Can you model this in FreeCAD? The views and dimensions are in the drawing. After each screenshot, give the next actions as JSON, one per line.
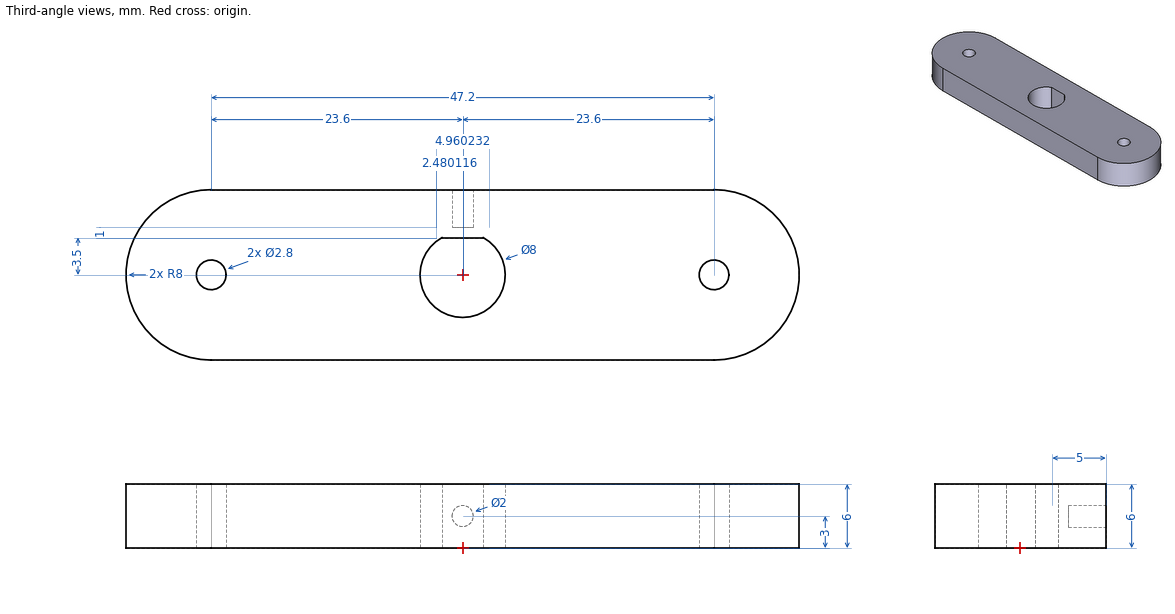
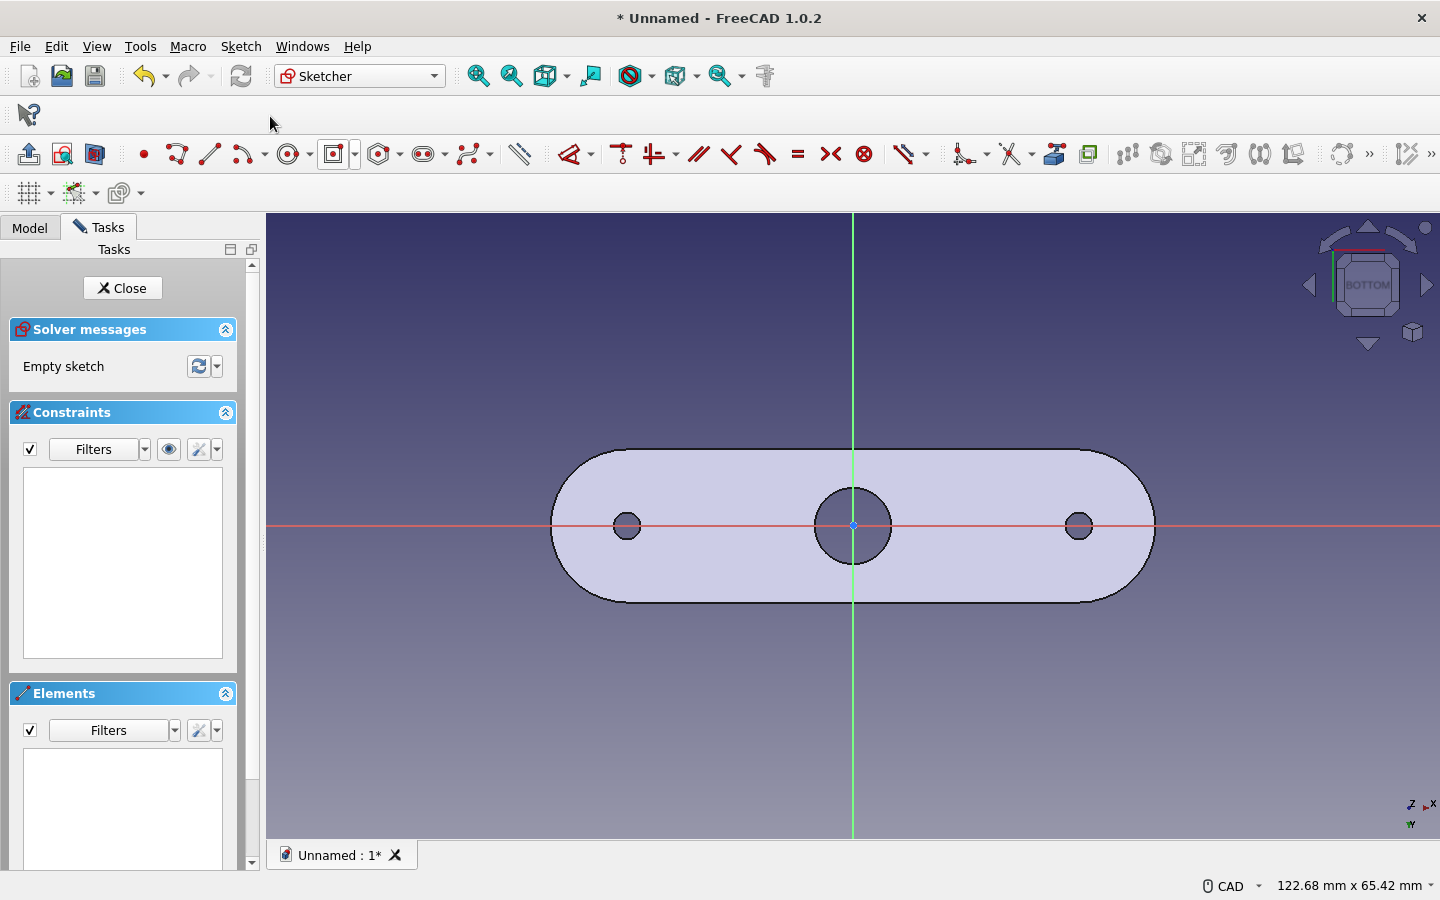
{"action": "scroll", "coordinate": [862, 550], "scroll_direction": "up", "scroll_amount": 11}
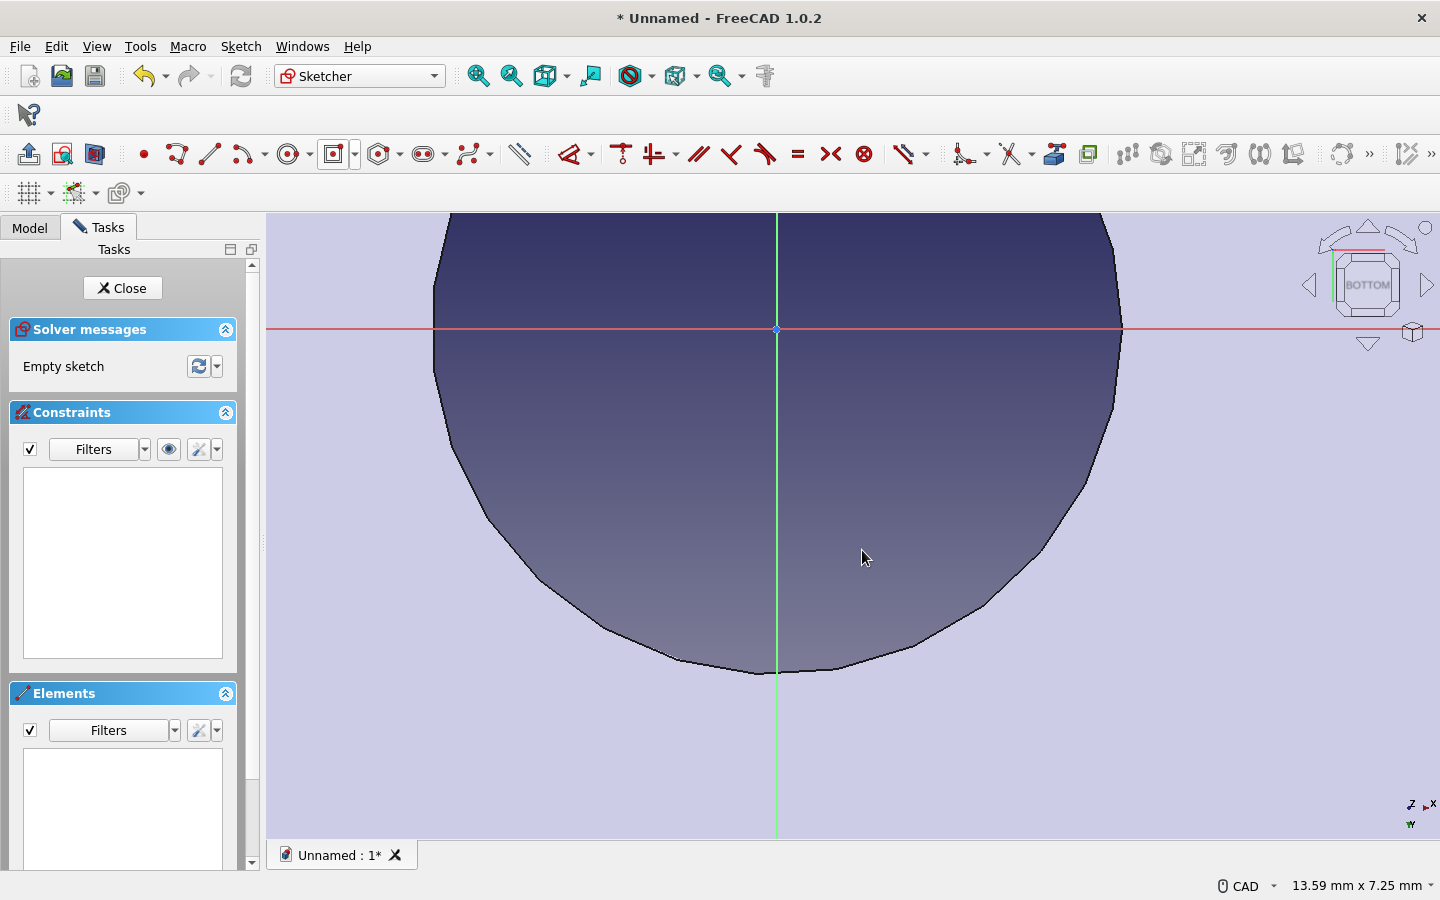
{"action": "left_click", "coordinate": [354, 154]}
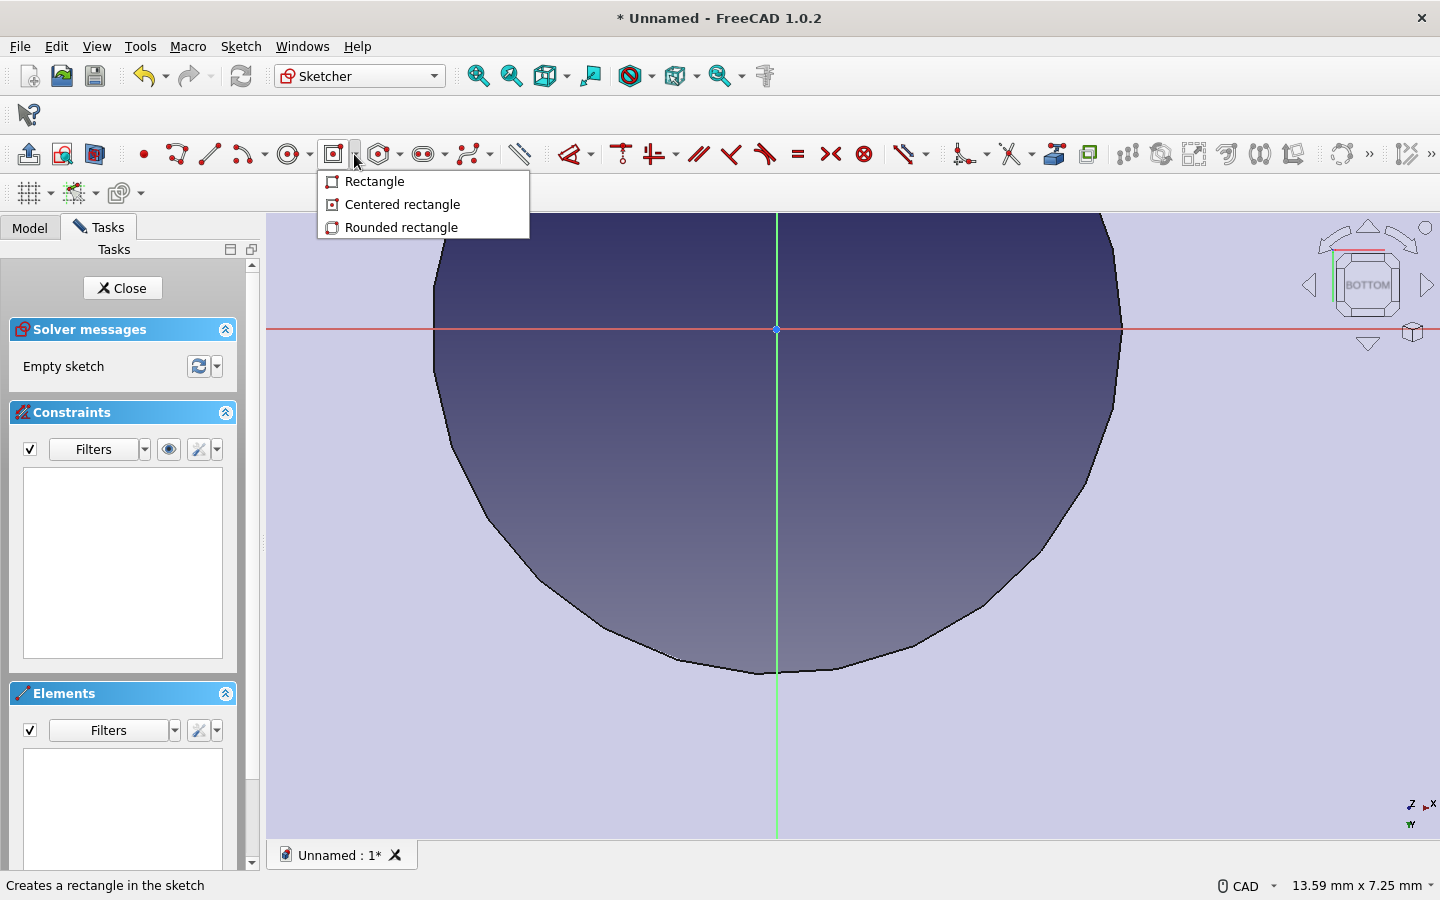
{"action": "left_click", "coordinate": [424, 182]}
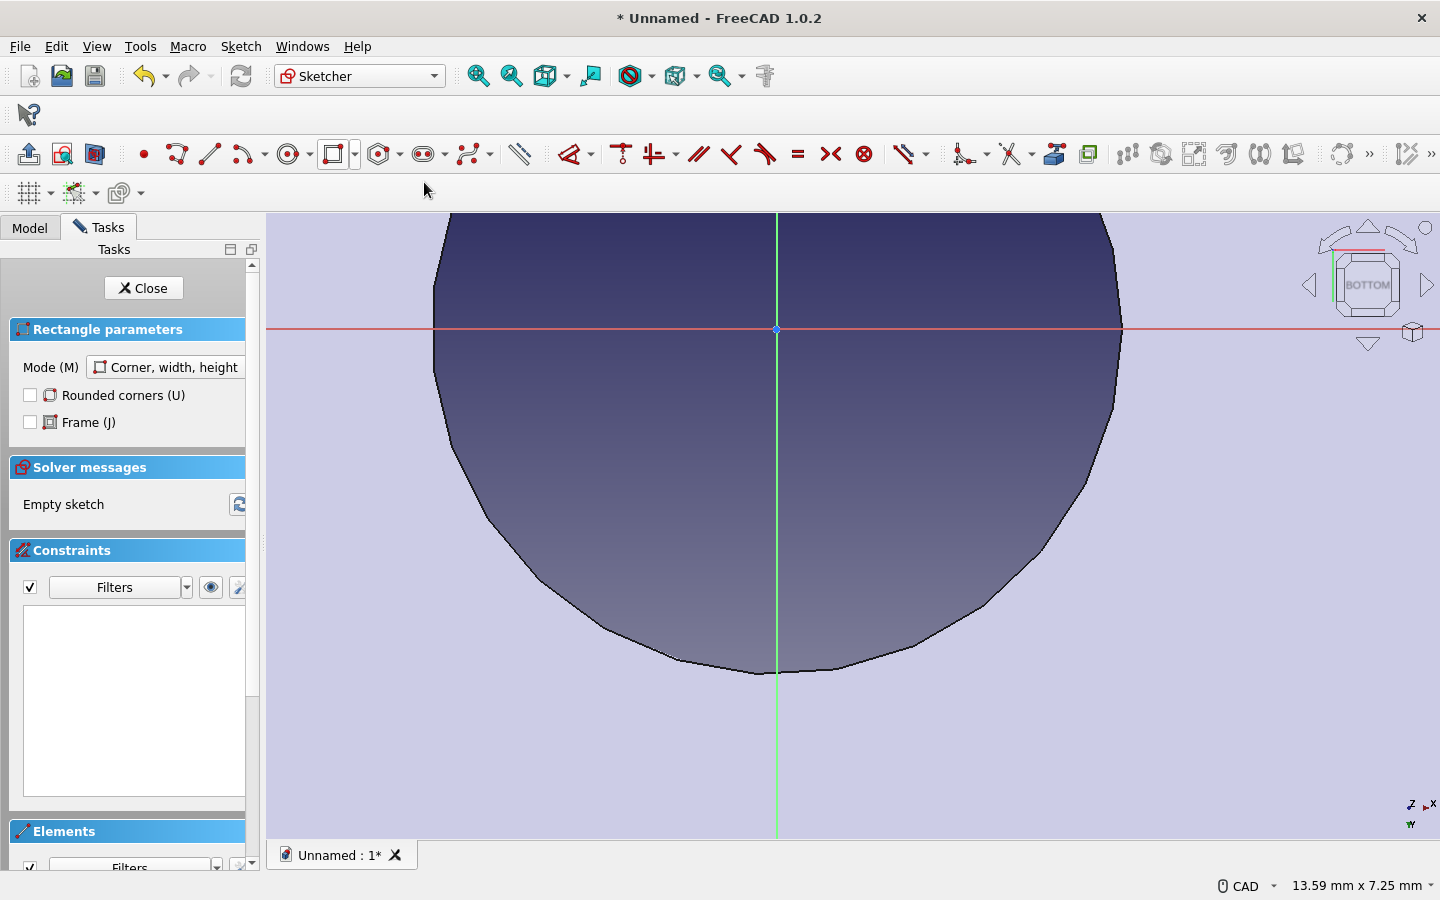
{"action": "left_click", "coordinate": [563, 631]}
{"action": "left_click", "coordinate": [991, 718]}
{"action": "key", "text": "Escape"}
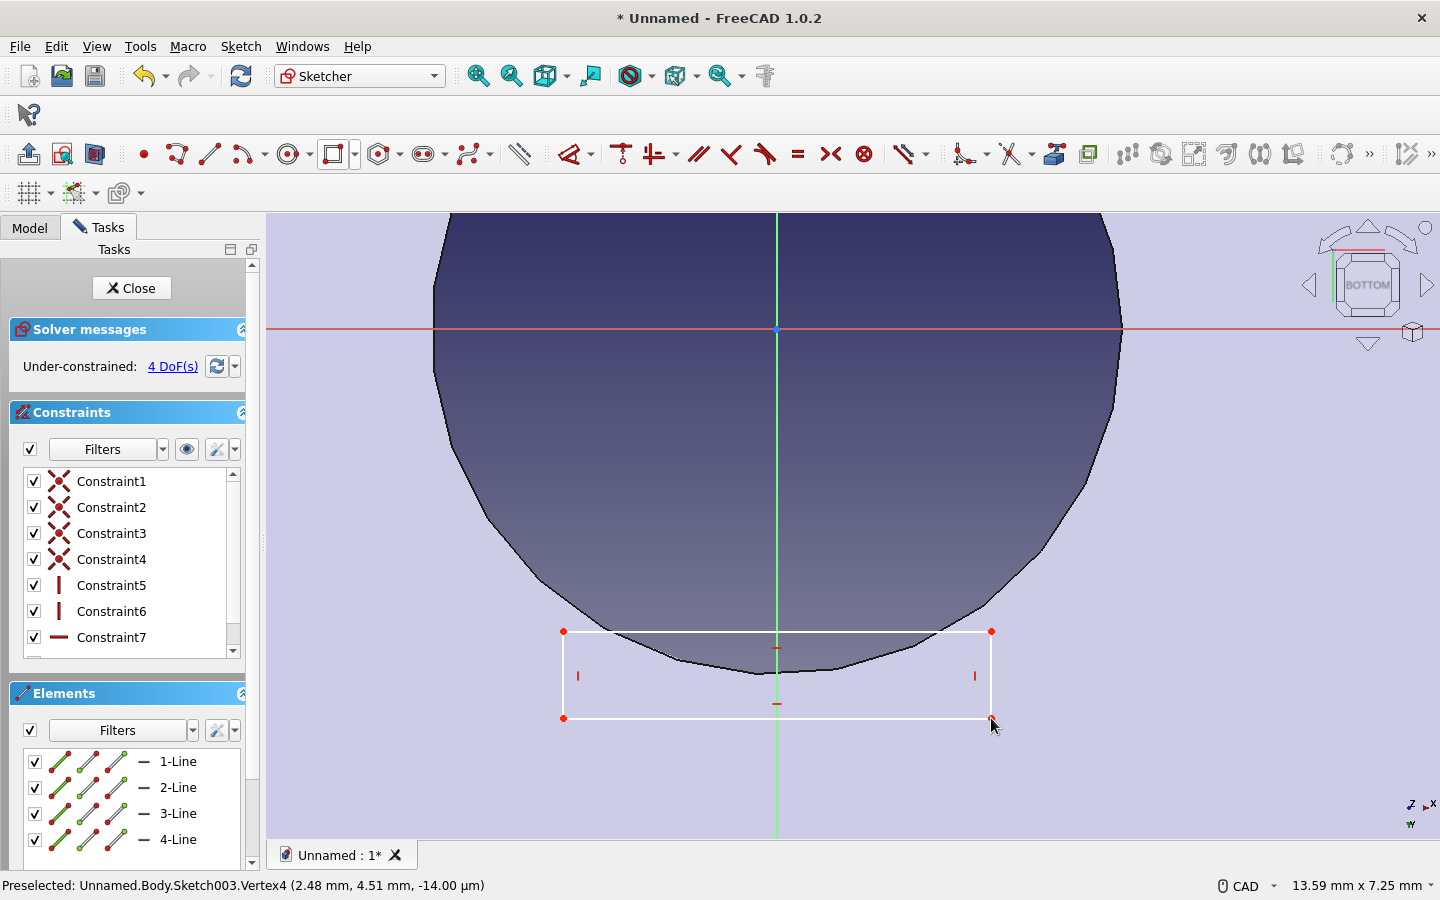
{"action": "left_click", "coordinate": [568, 154]}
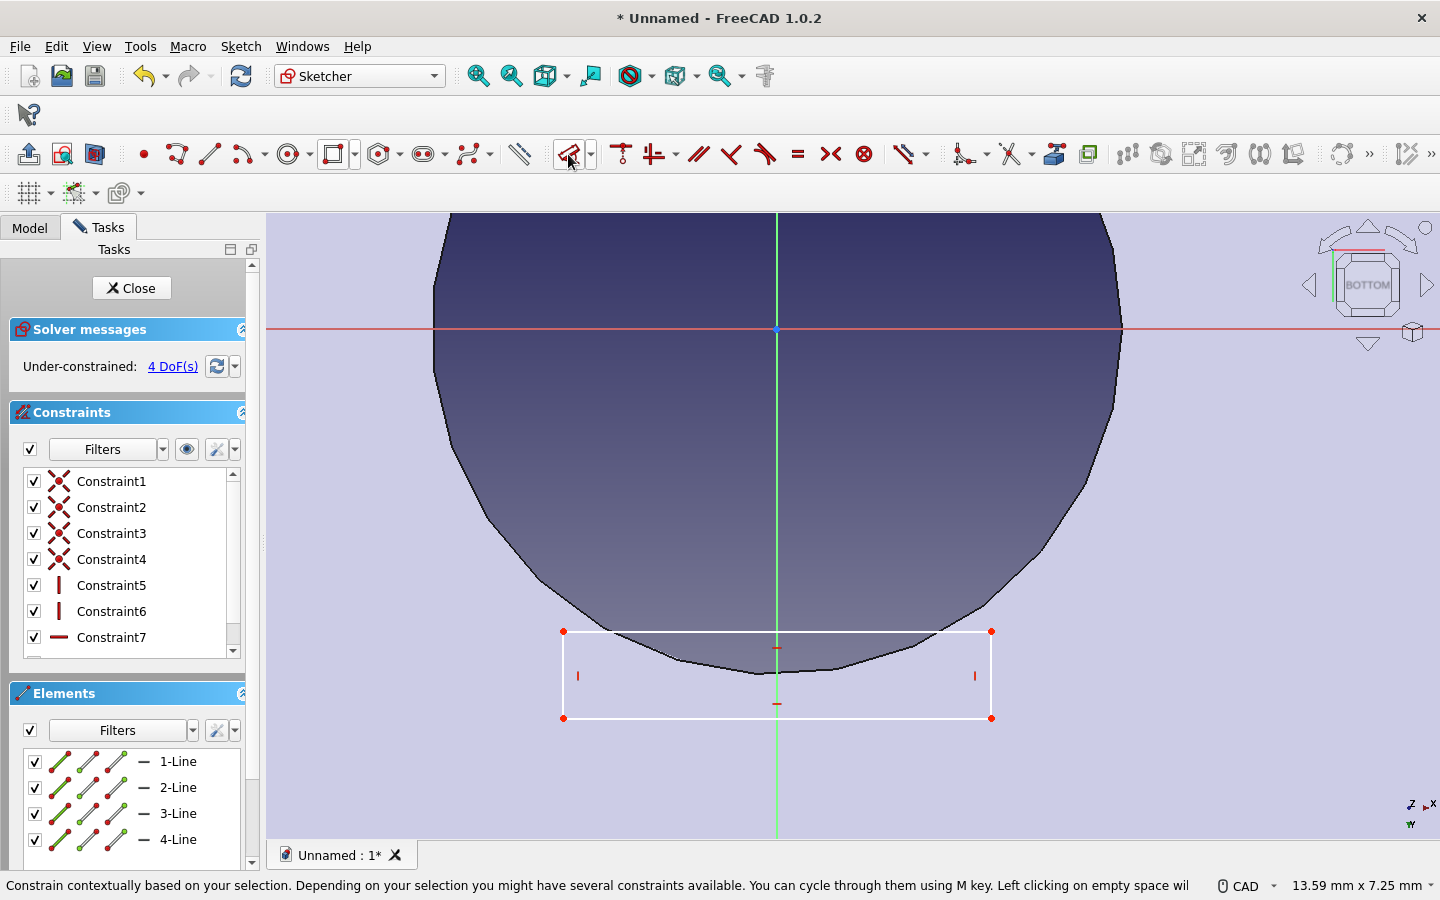
{"action": "left_click", "coordinate": [563, 658]}
{"action": "left_click", "coordinate": [529, 676]}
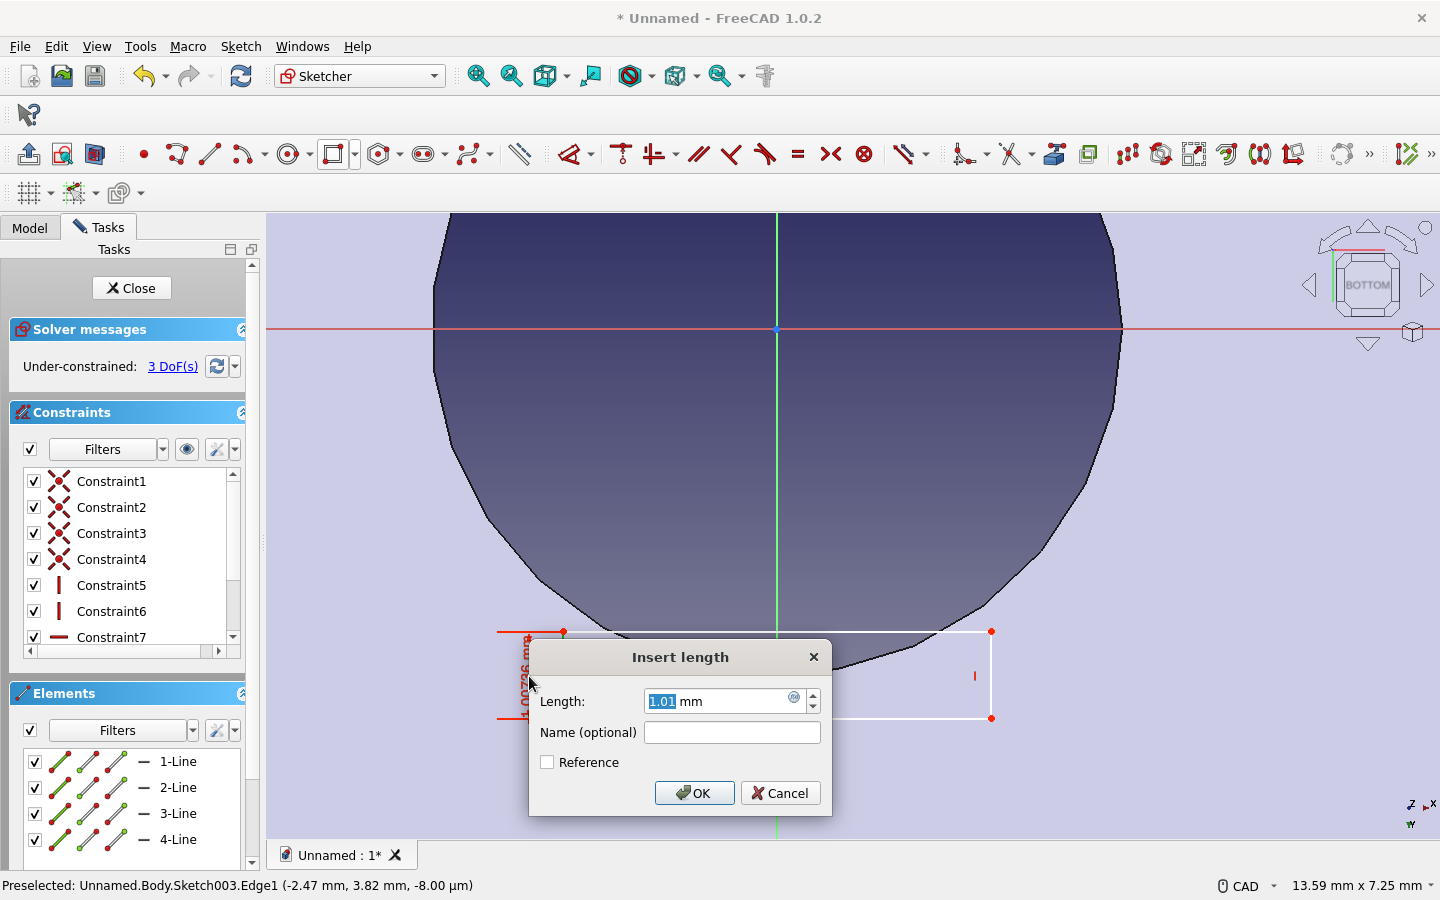
{"action": "type", "text": "1"}
{"action": "key", "text": "Return"}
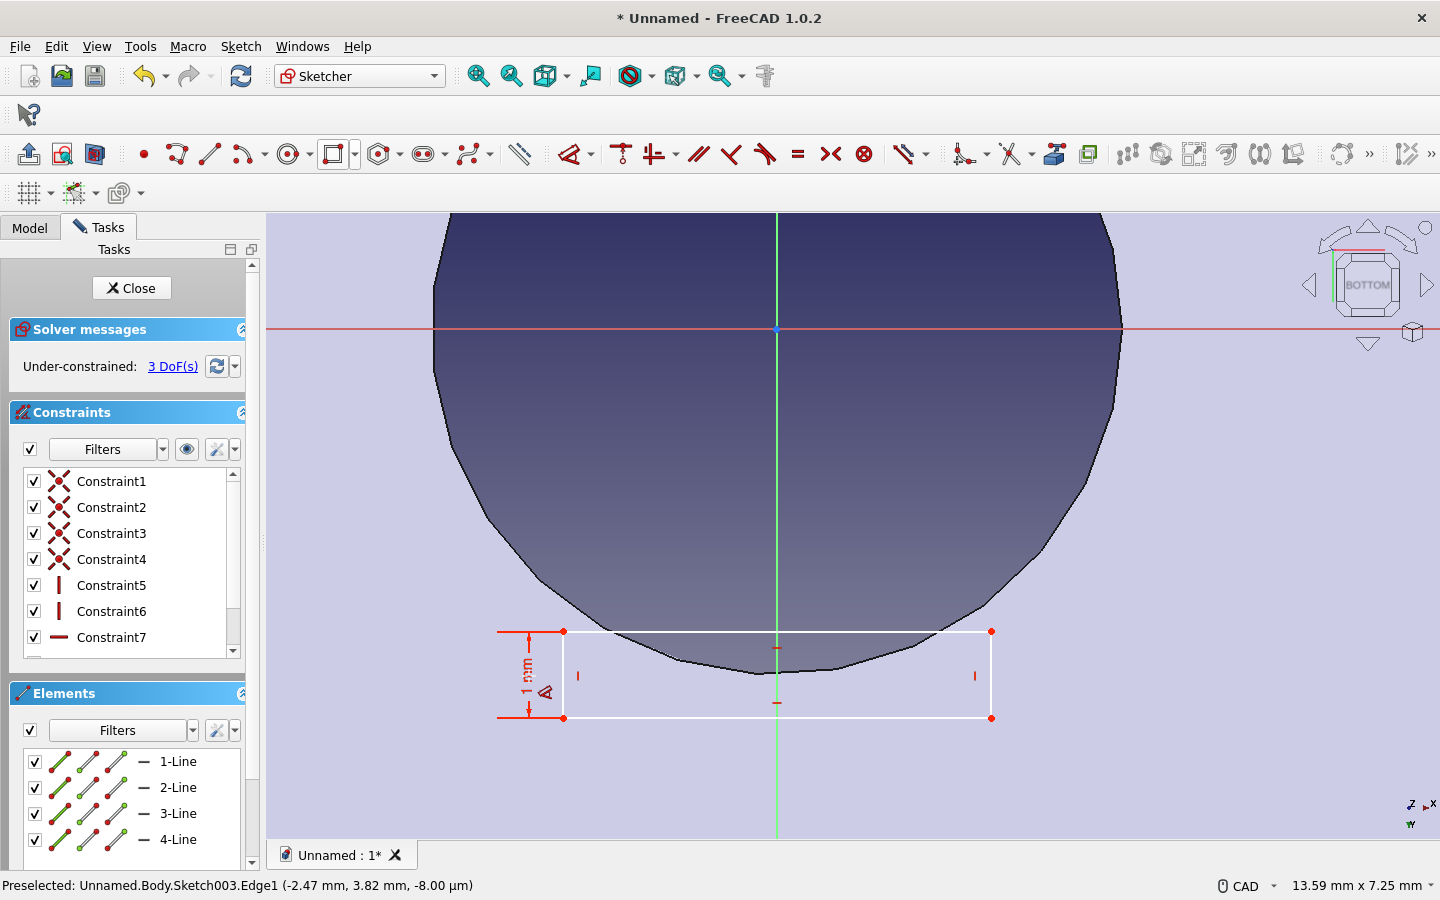
{"action": "left_click", "coordinate": [563, 632]}
{"action": "left_click", "coordinate": [529, 481]}